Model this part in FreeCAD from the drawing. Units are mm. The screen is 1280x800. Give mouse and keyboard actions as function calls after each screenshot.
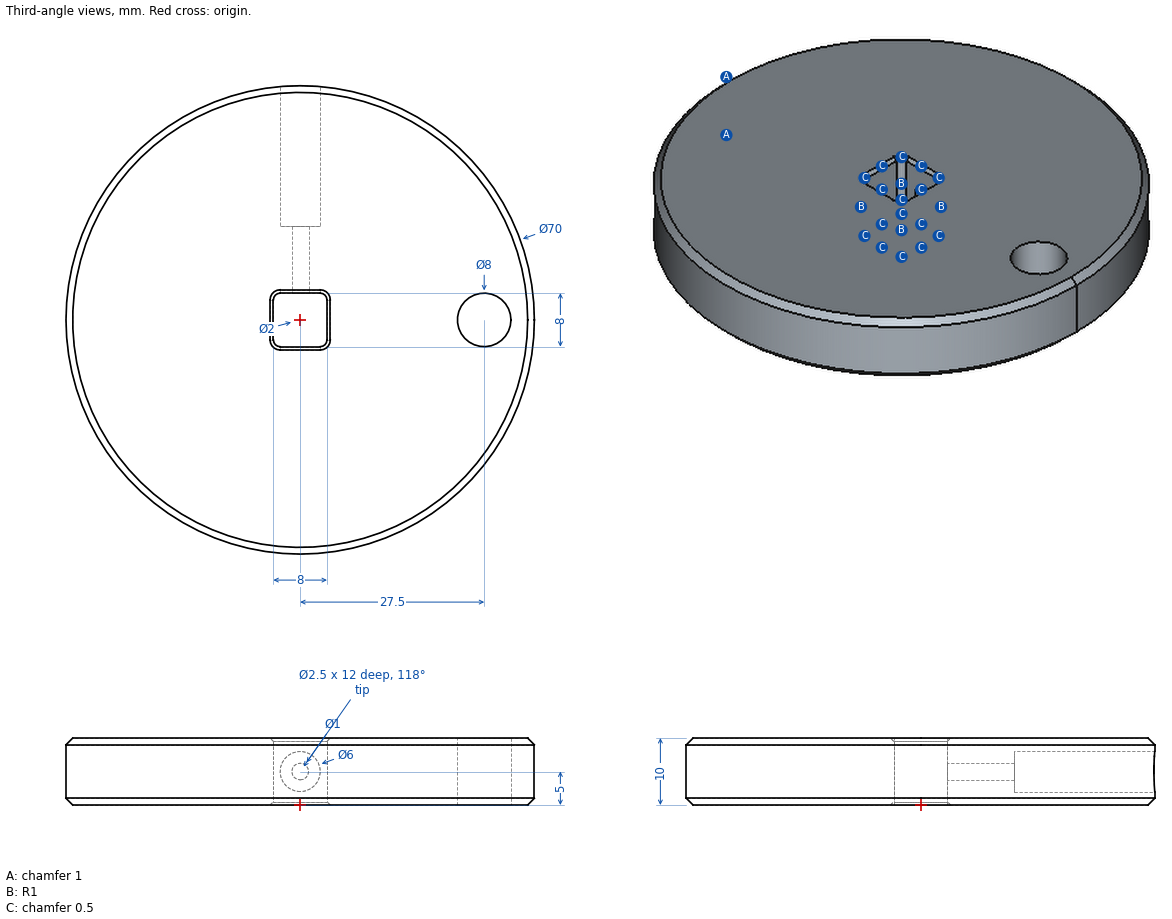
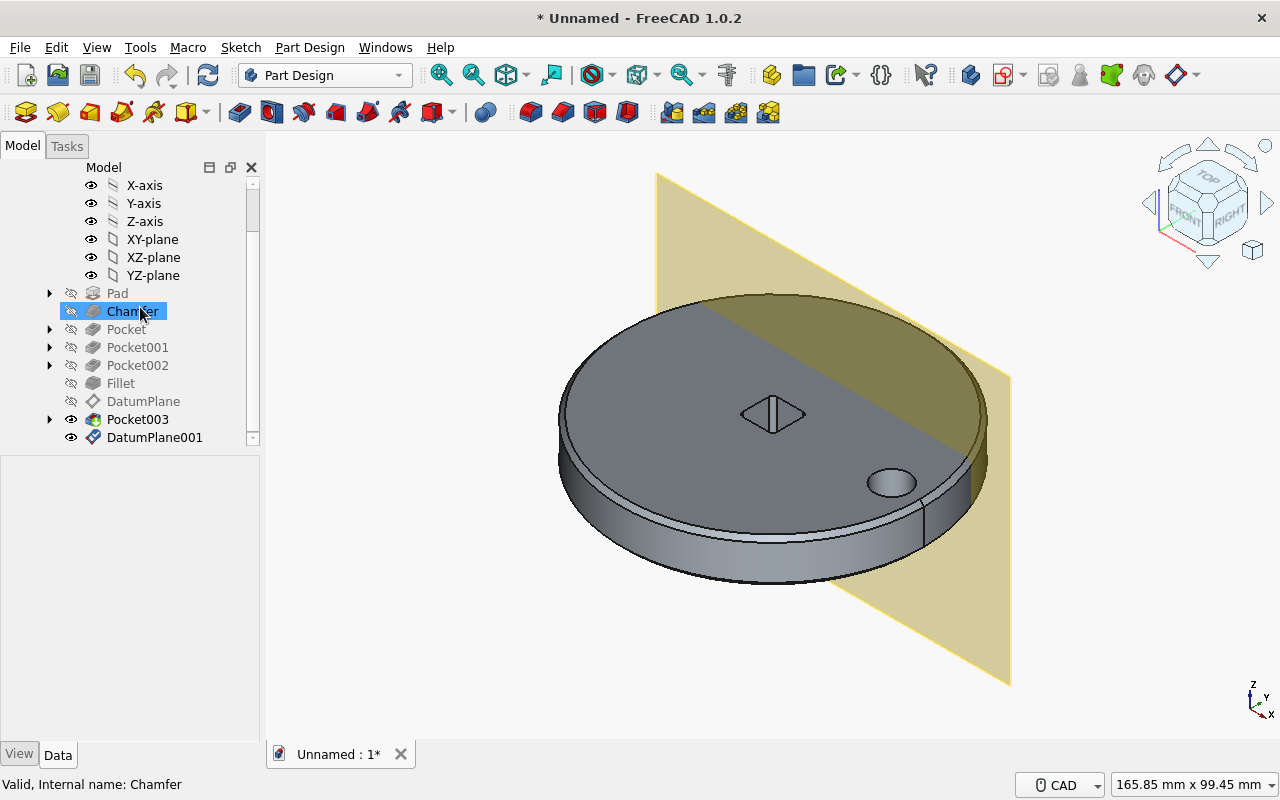
click(116, 437)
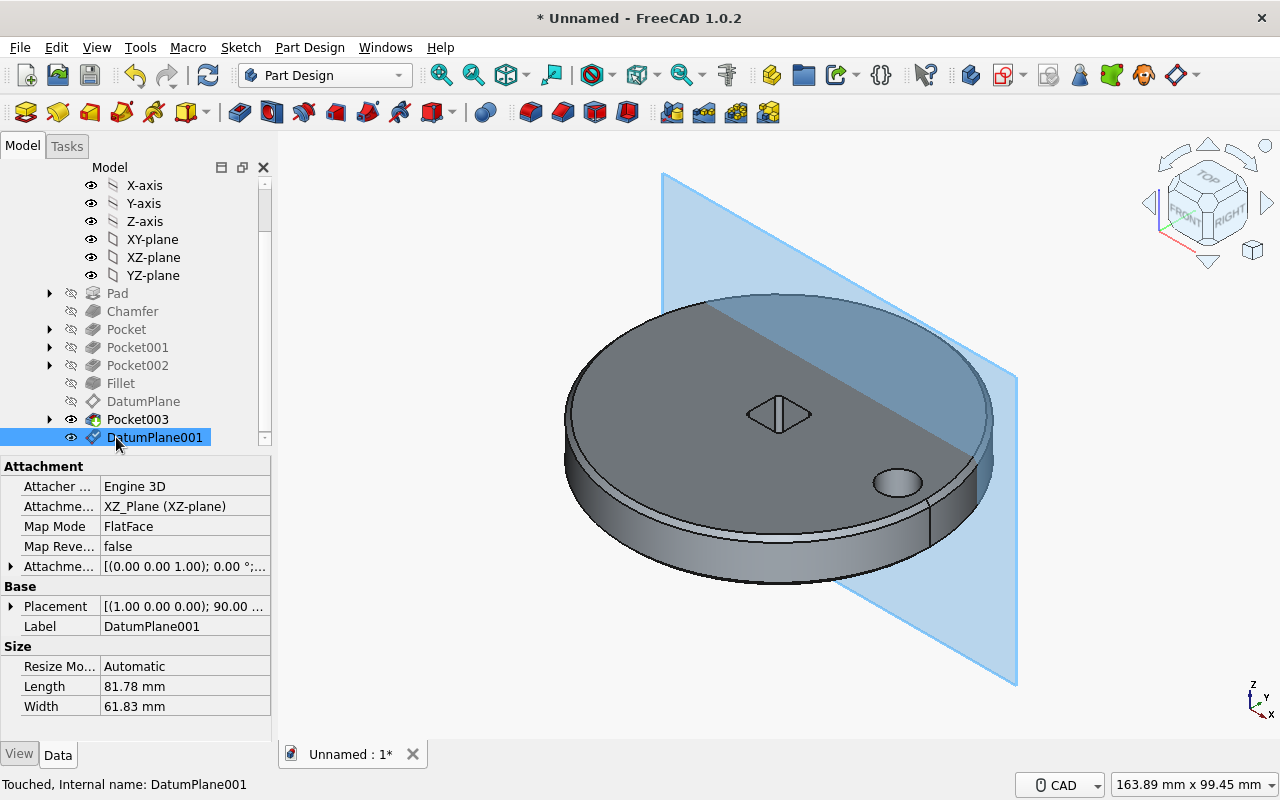
click(1004, 76)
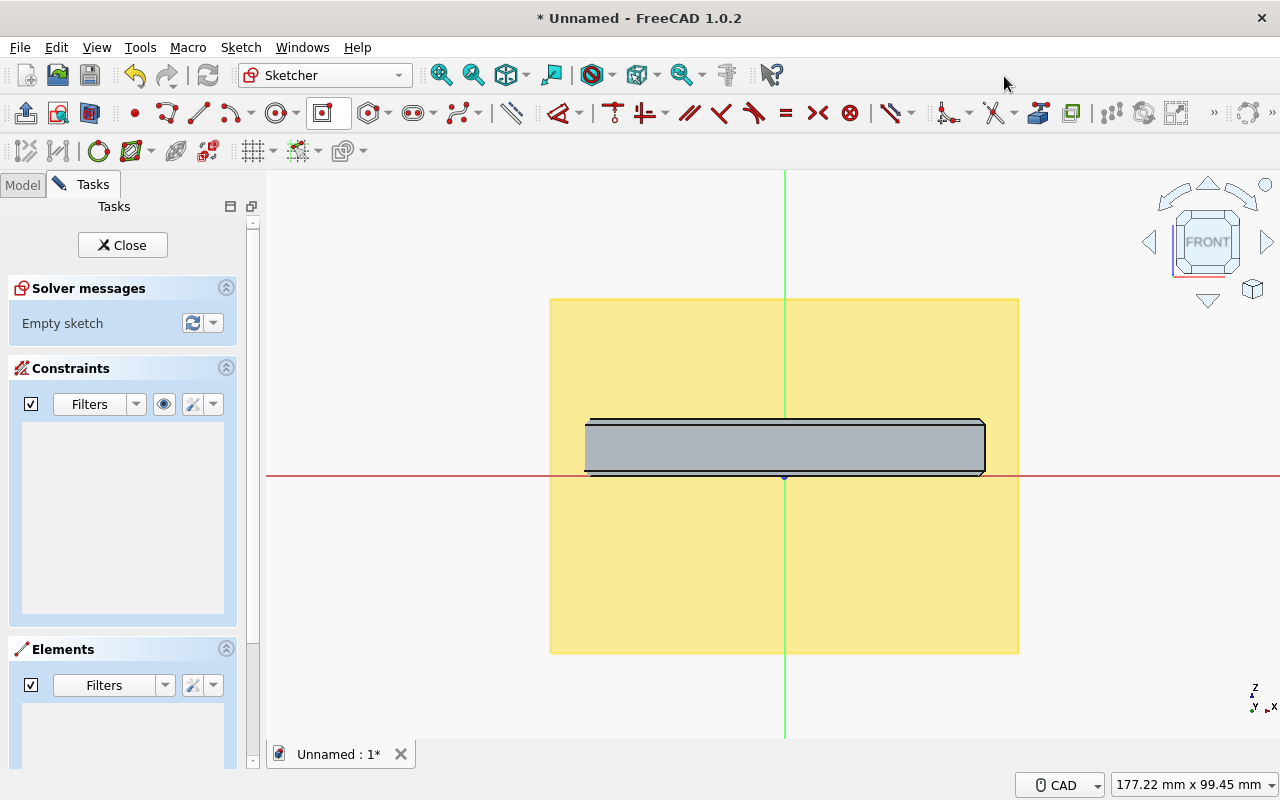
click(90, 114)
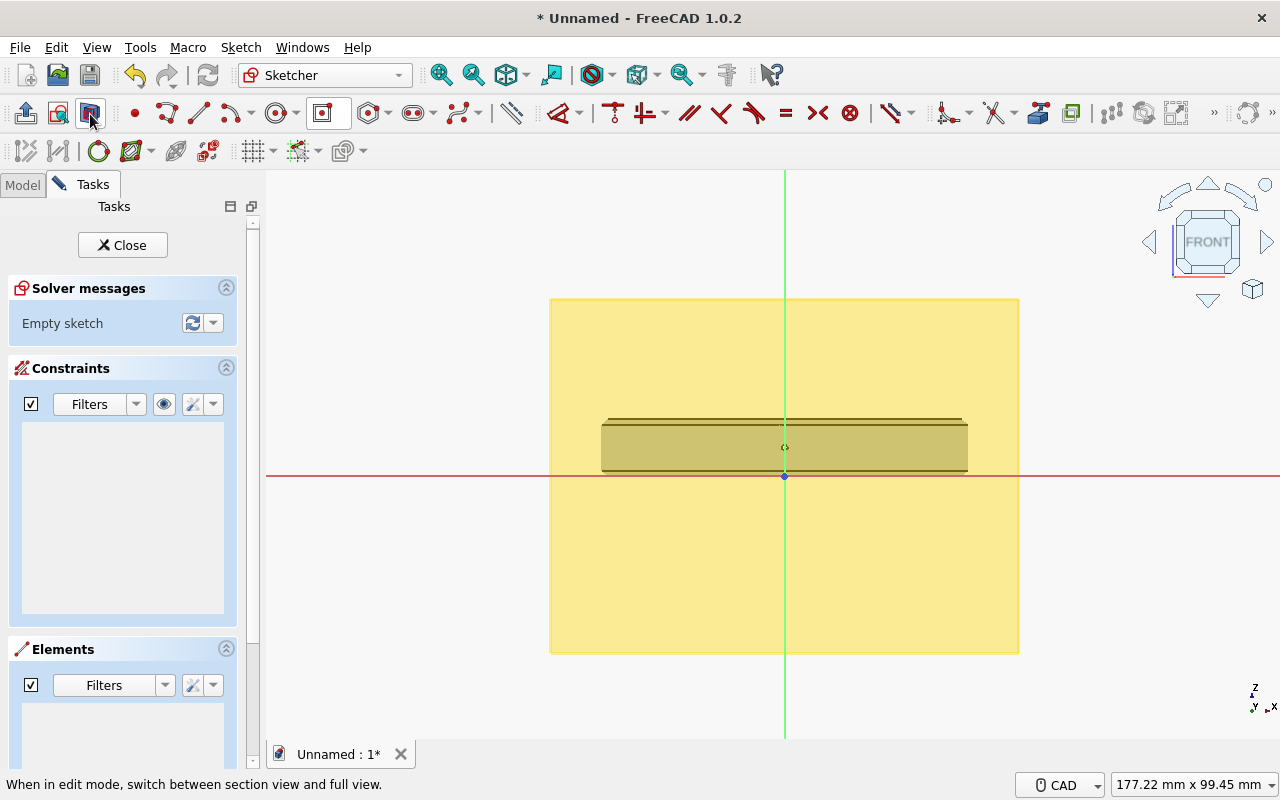
scroll(797, 453, up, 10)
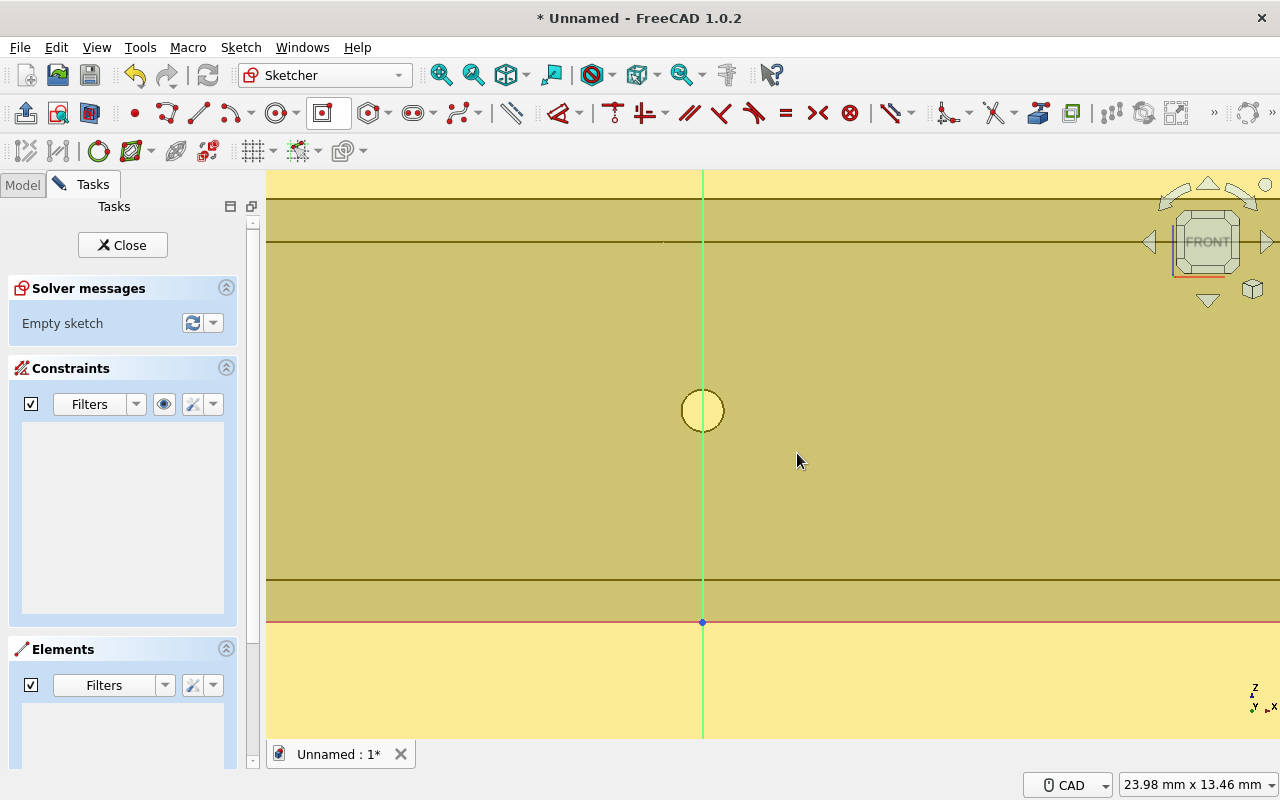
click(276, 114)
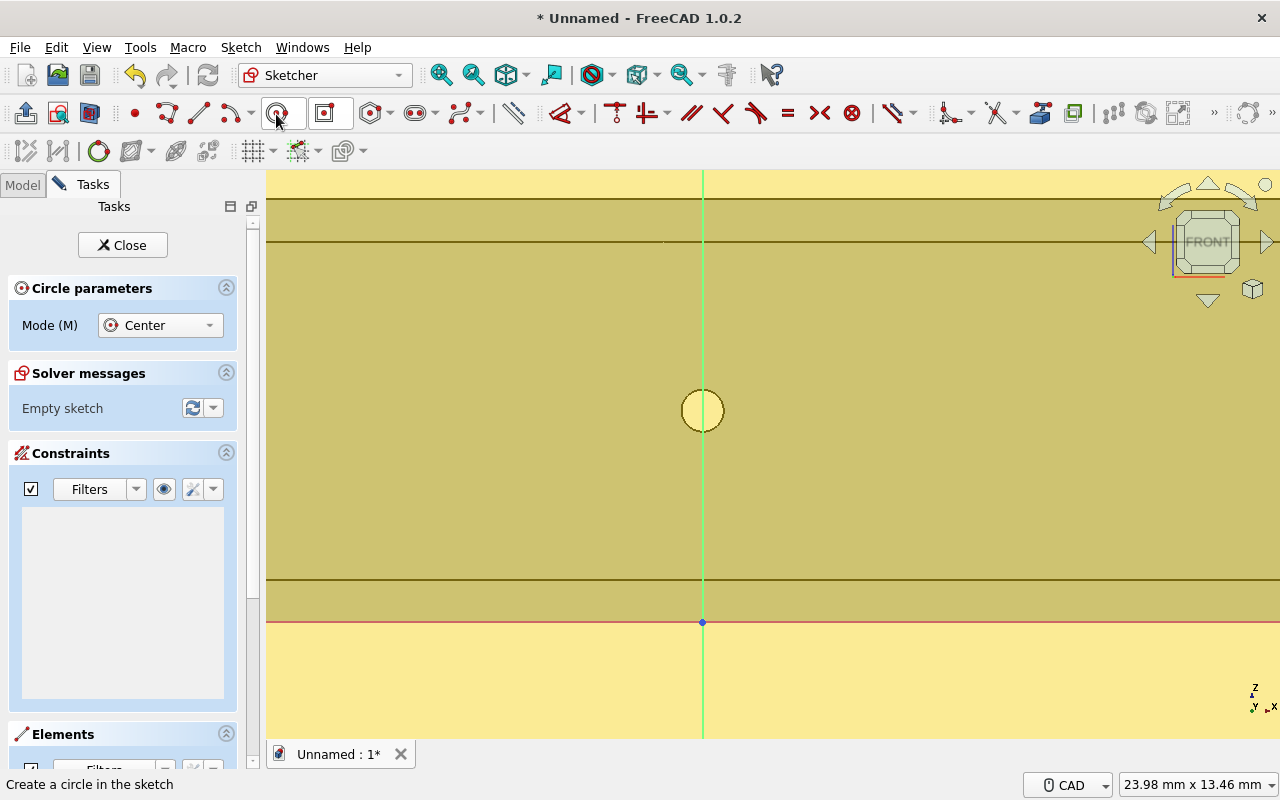
click(703, 411)
click(792, 321)
key(Escape)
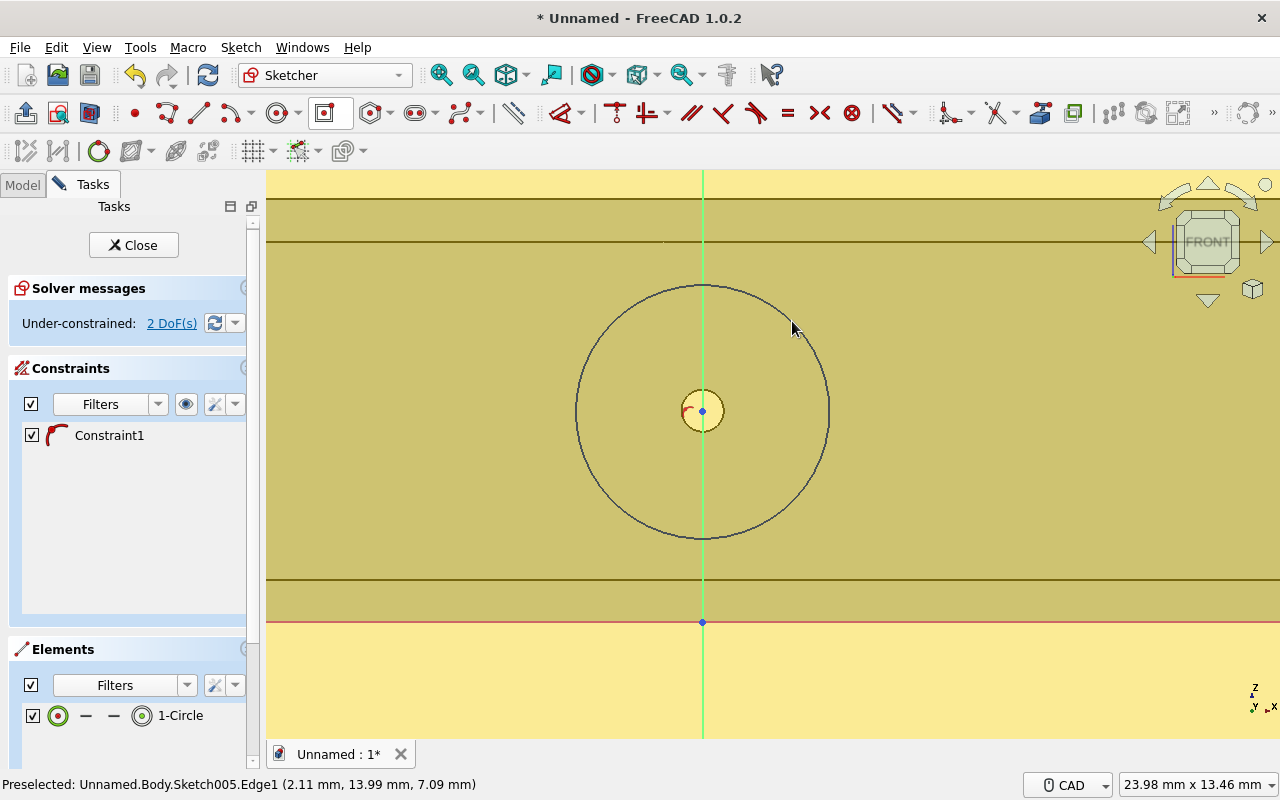
click(560, 114)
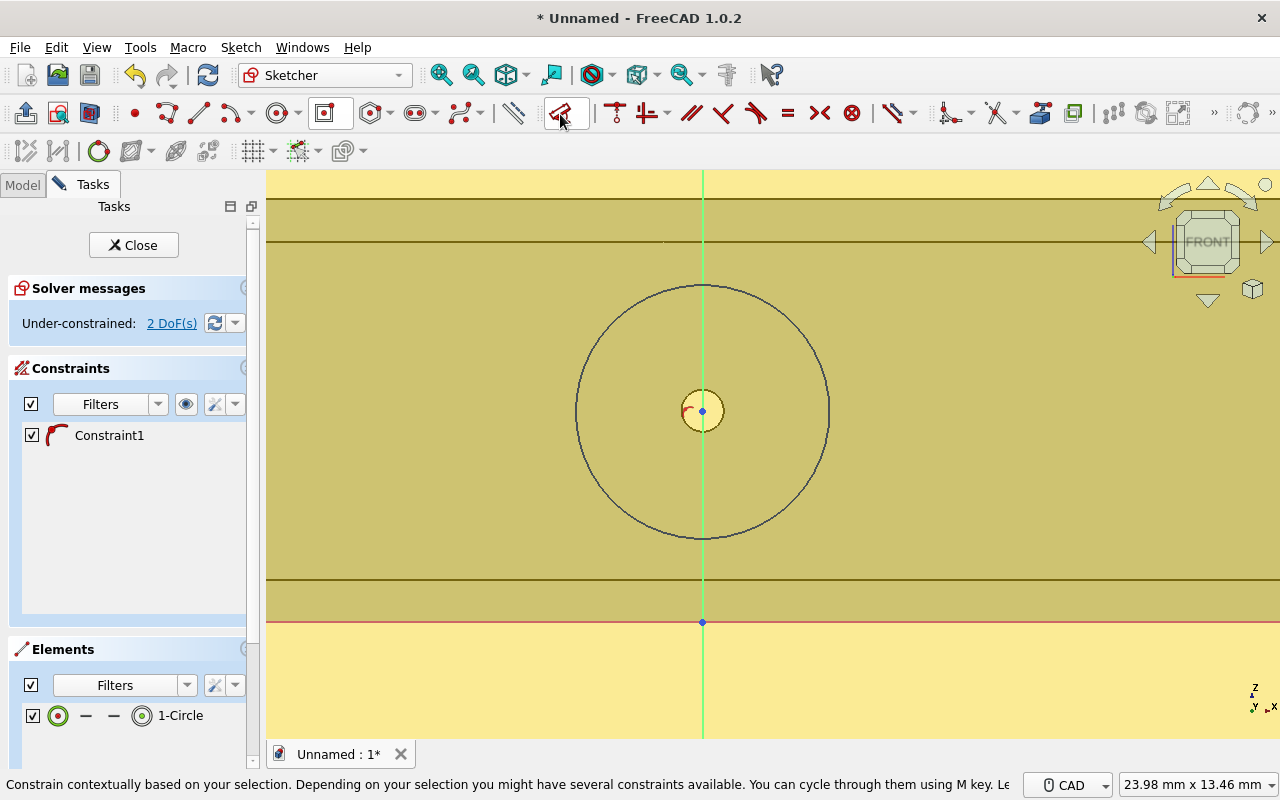
click(792, 322)
click(815, 299)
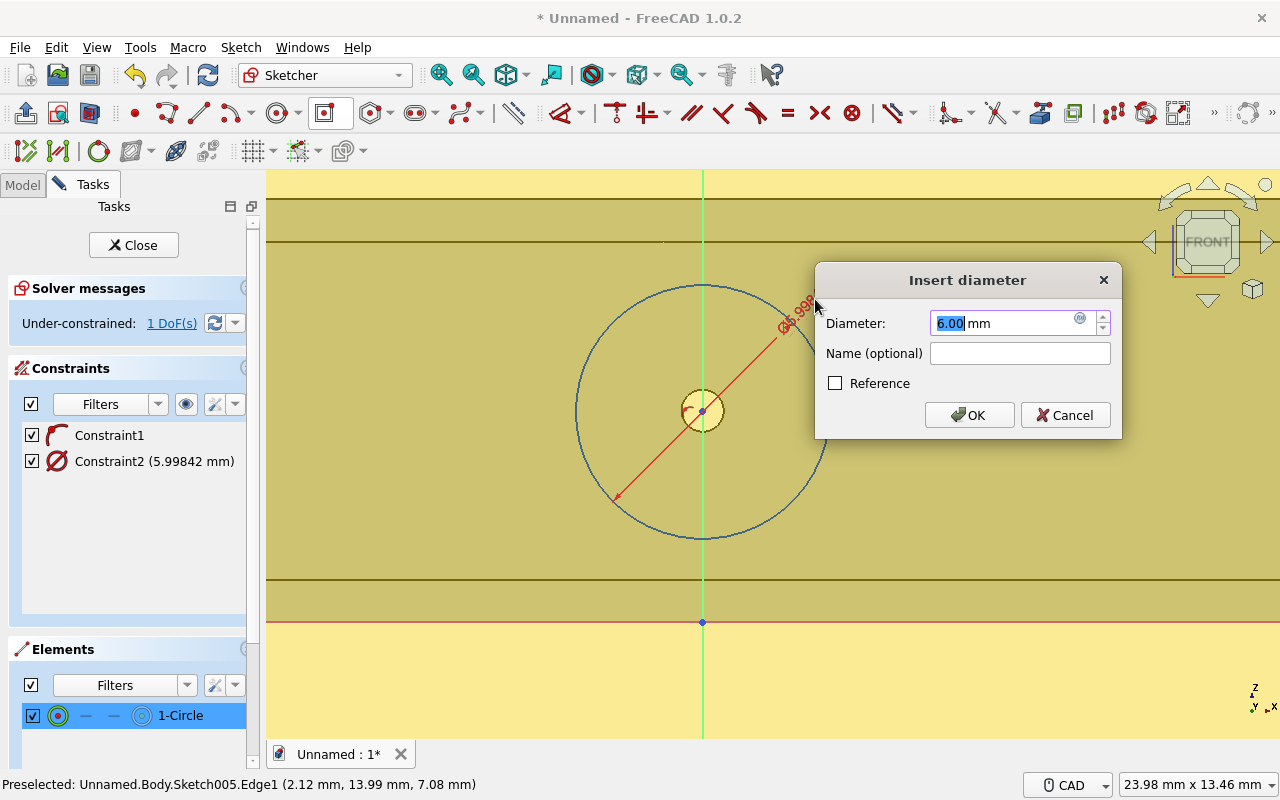
text(6)
key(Return)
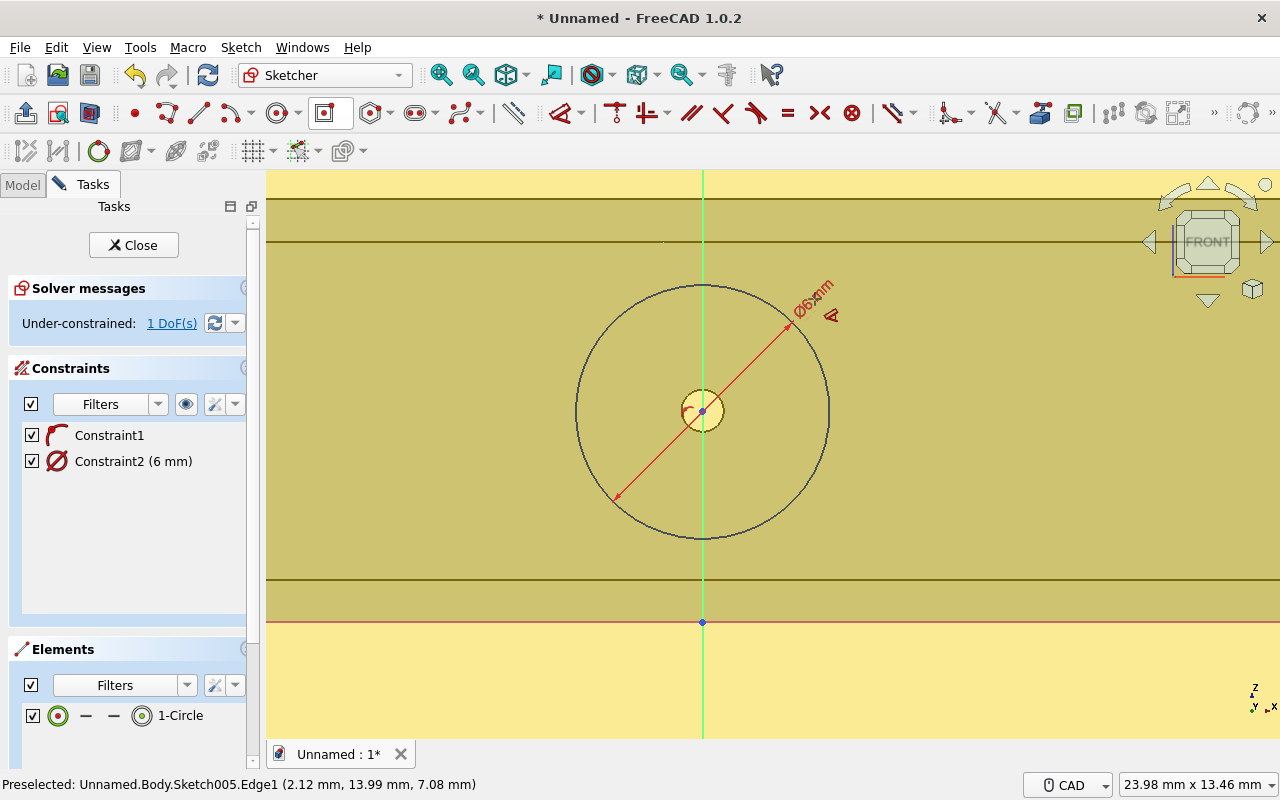
click(703, 412)
click(737, 517)